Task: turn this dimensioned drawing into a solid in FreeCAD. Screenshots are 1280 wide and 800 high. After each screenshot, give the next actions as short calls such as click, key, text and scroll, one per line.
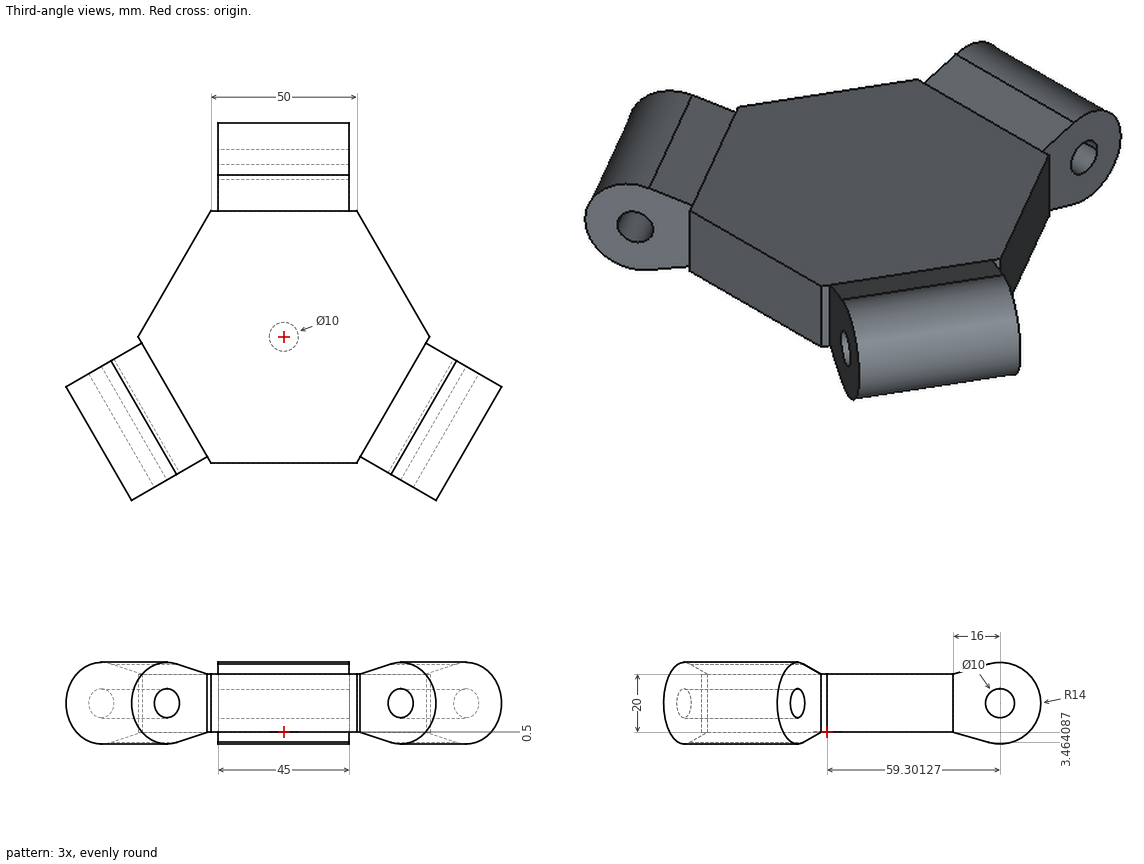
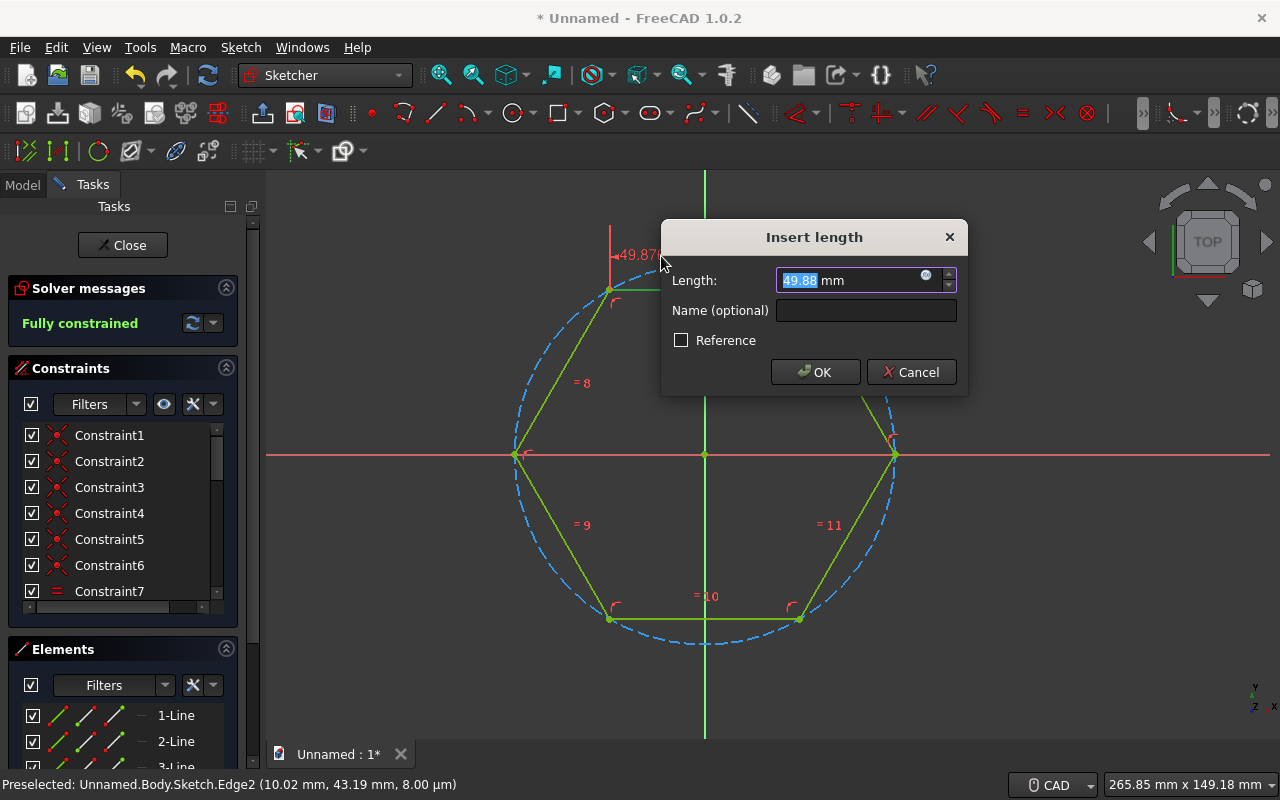
text(50)
key(Return)
key(Escape)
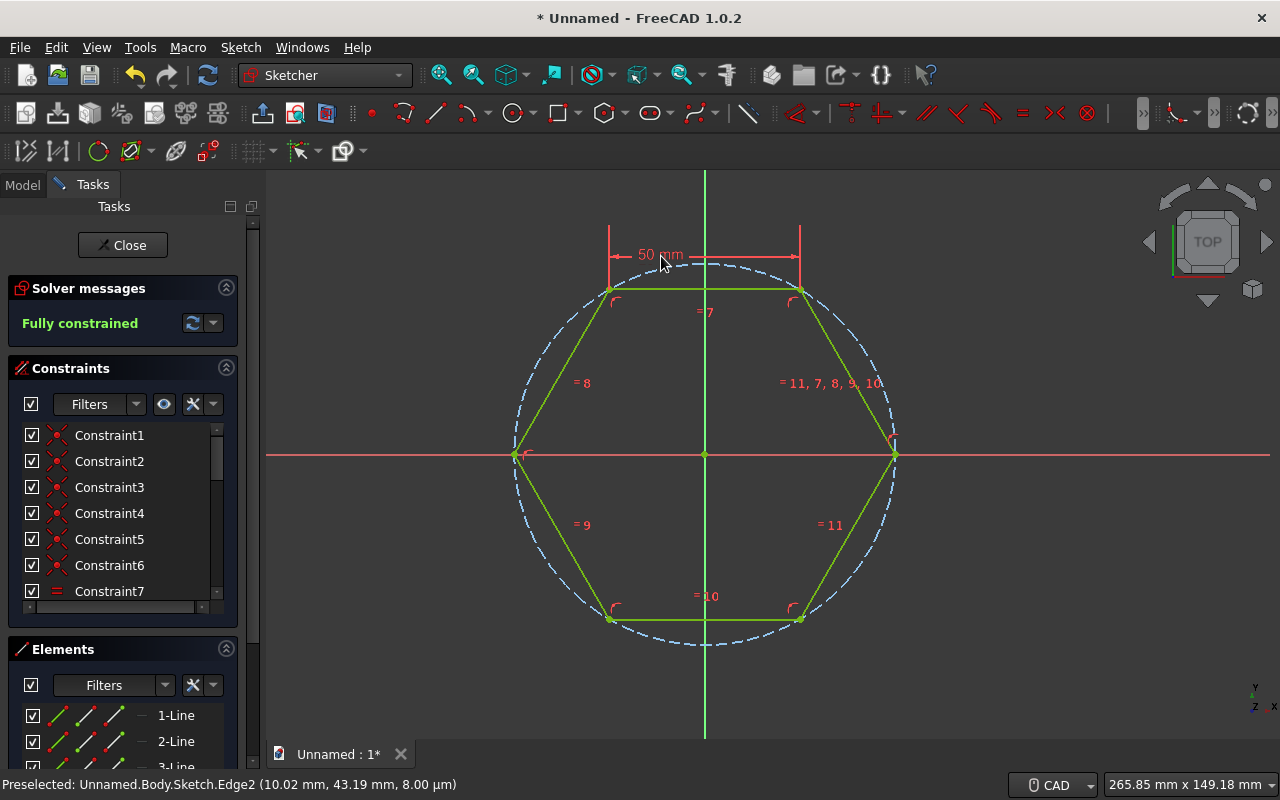
click(123, 245)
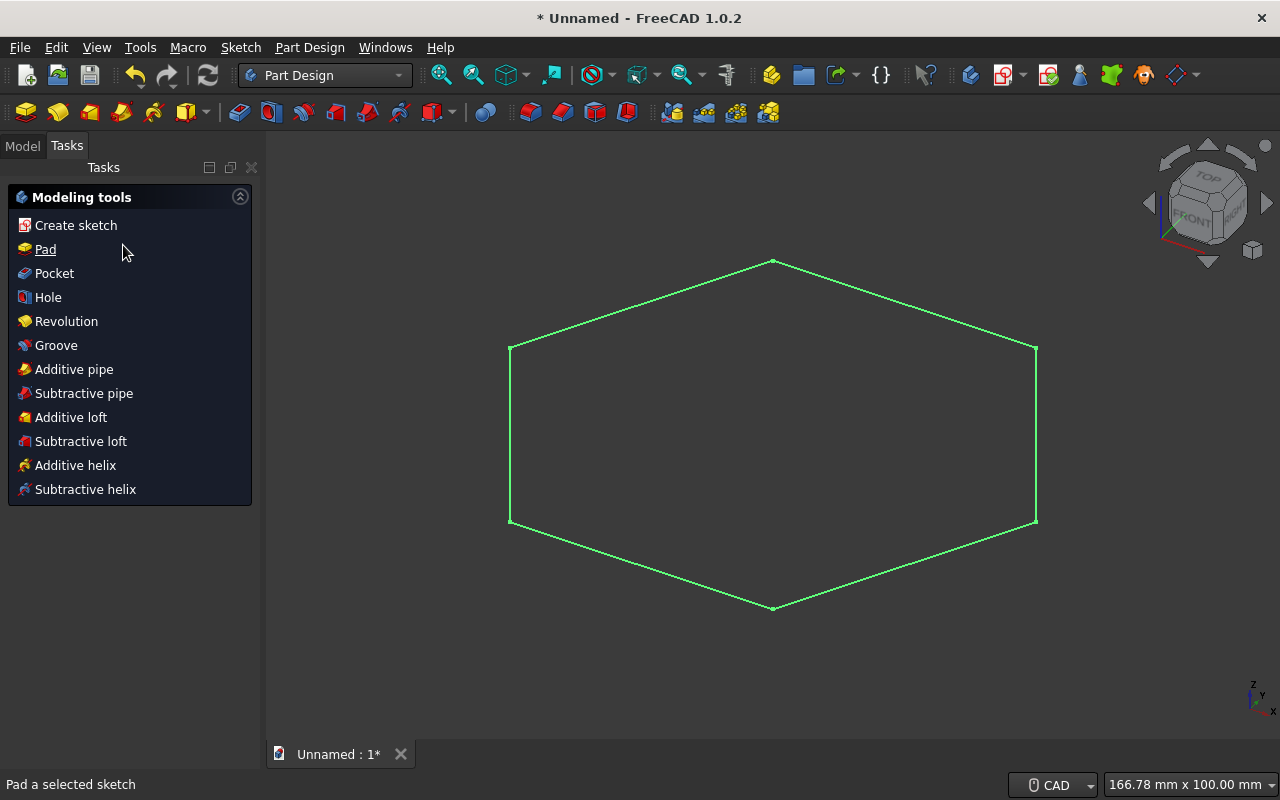
click(26, 112)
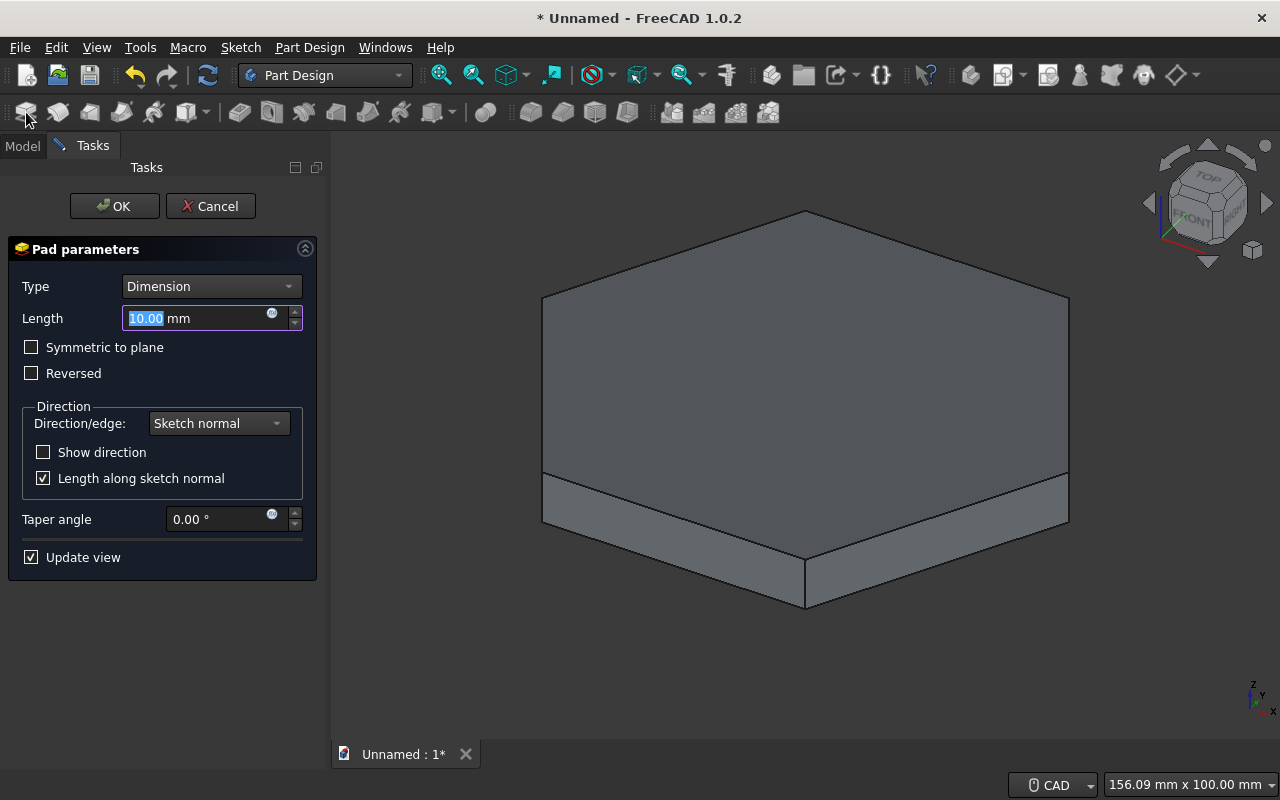
text(20)
key(Tab)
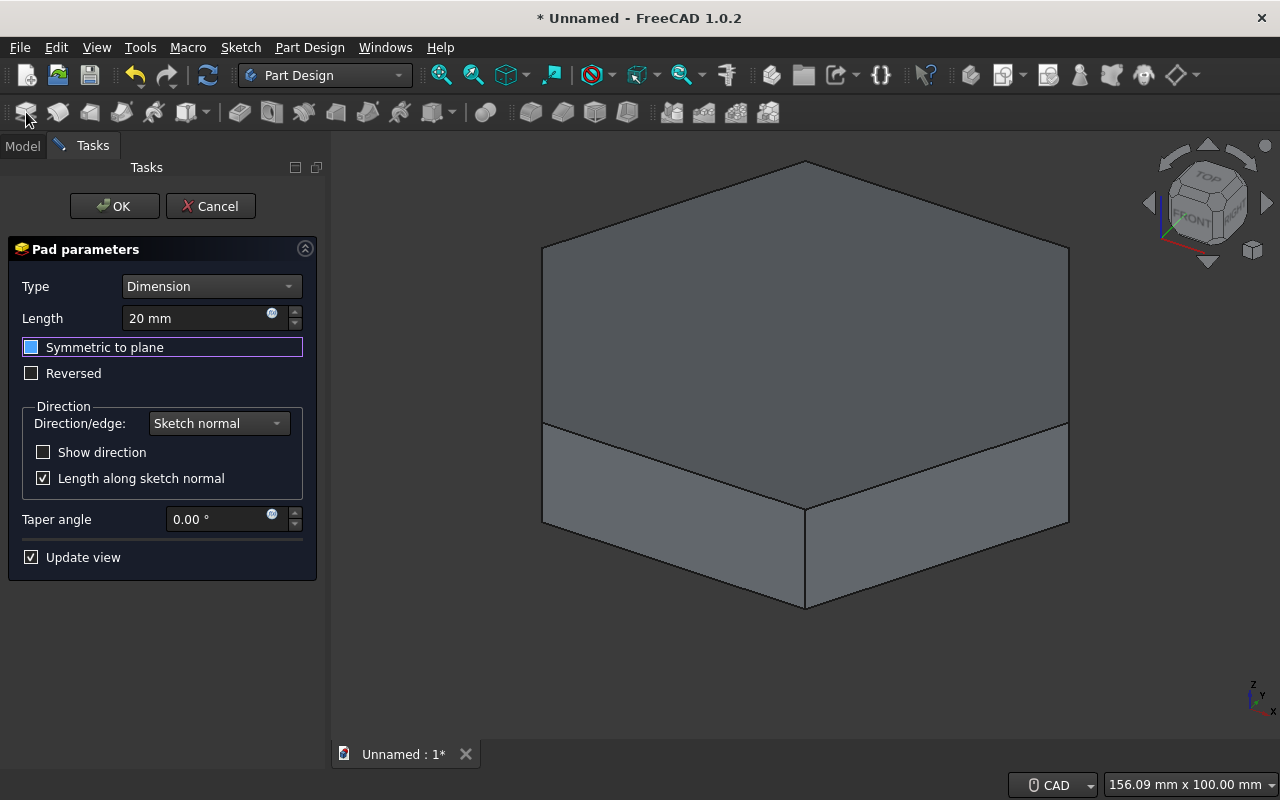
click(115, 206)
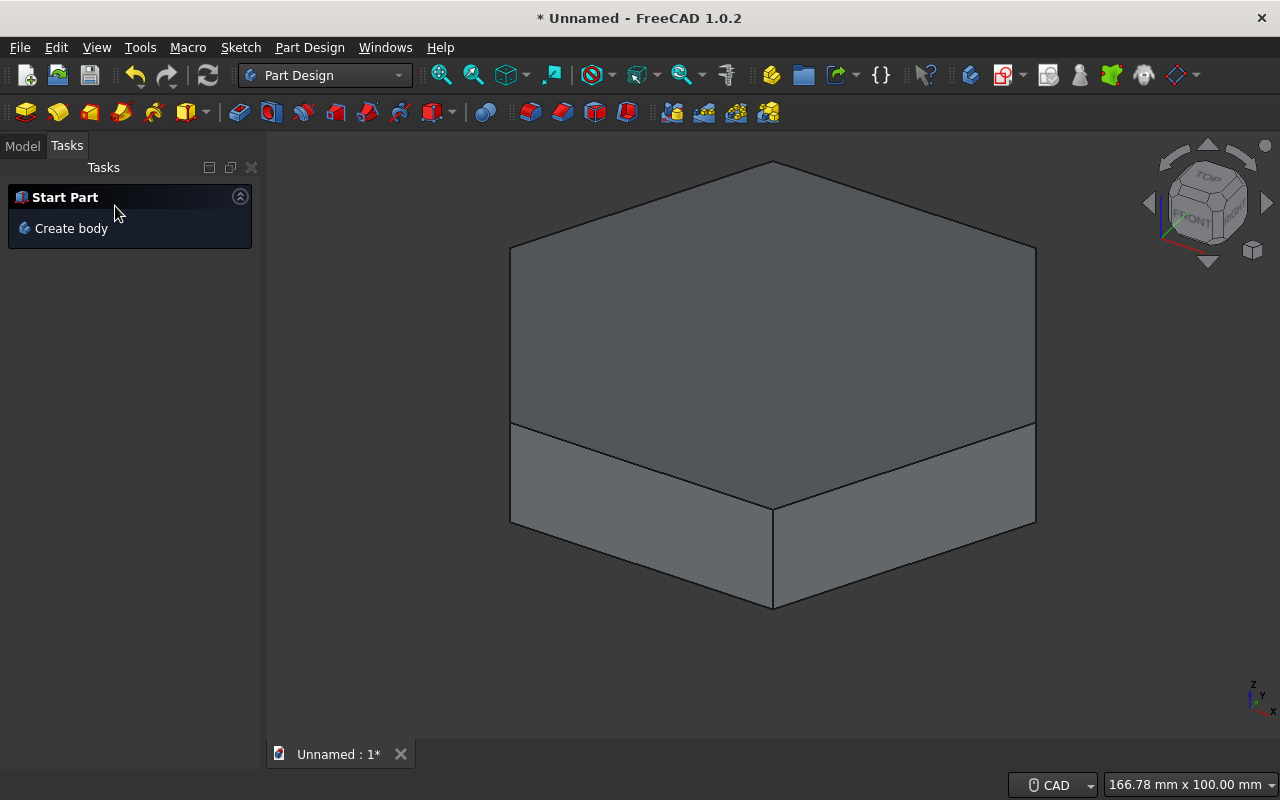
click(442, 76)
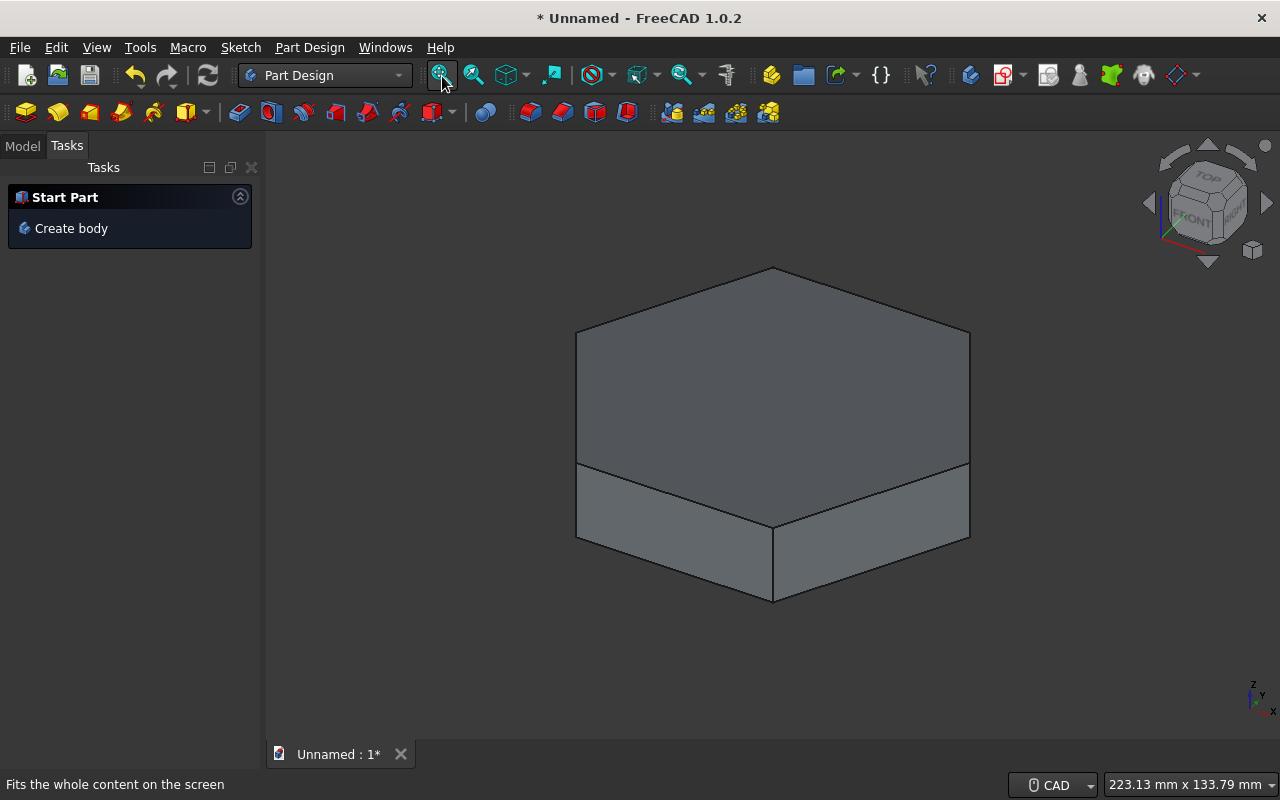
click(1004, 76)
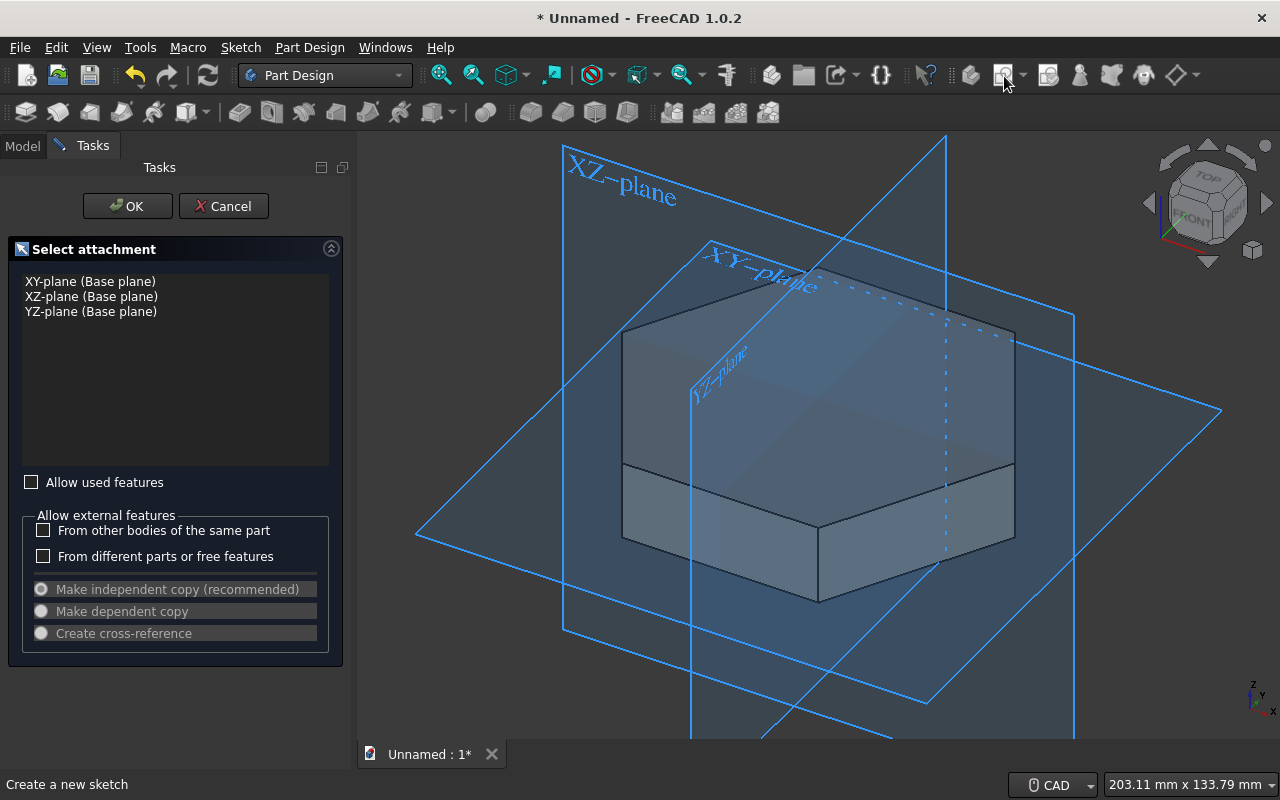
click(82, 312)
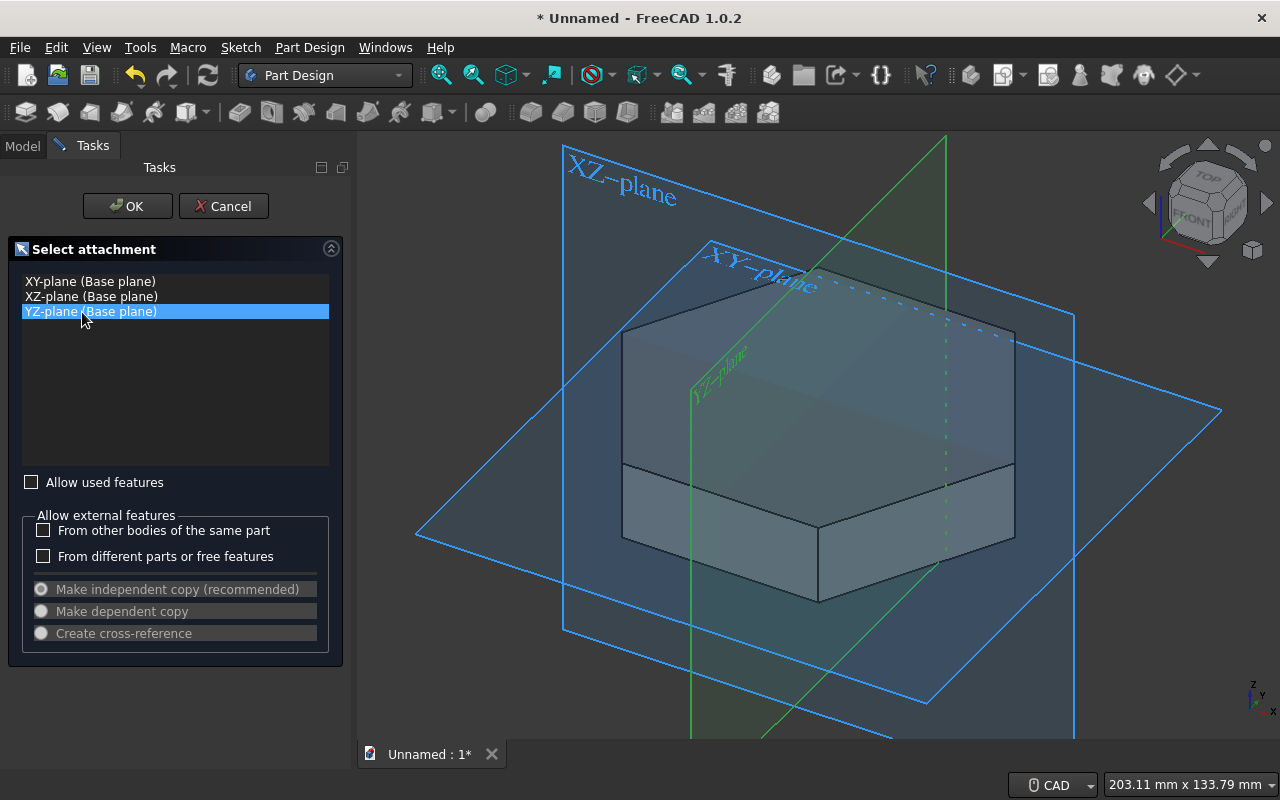
click(128, 206)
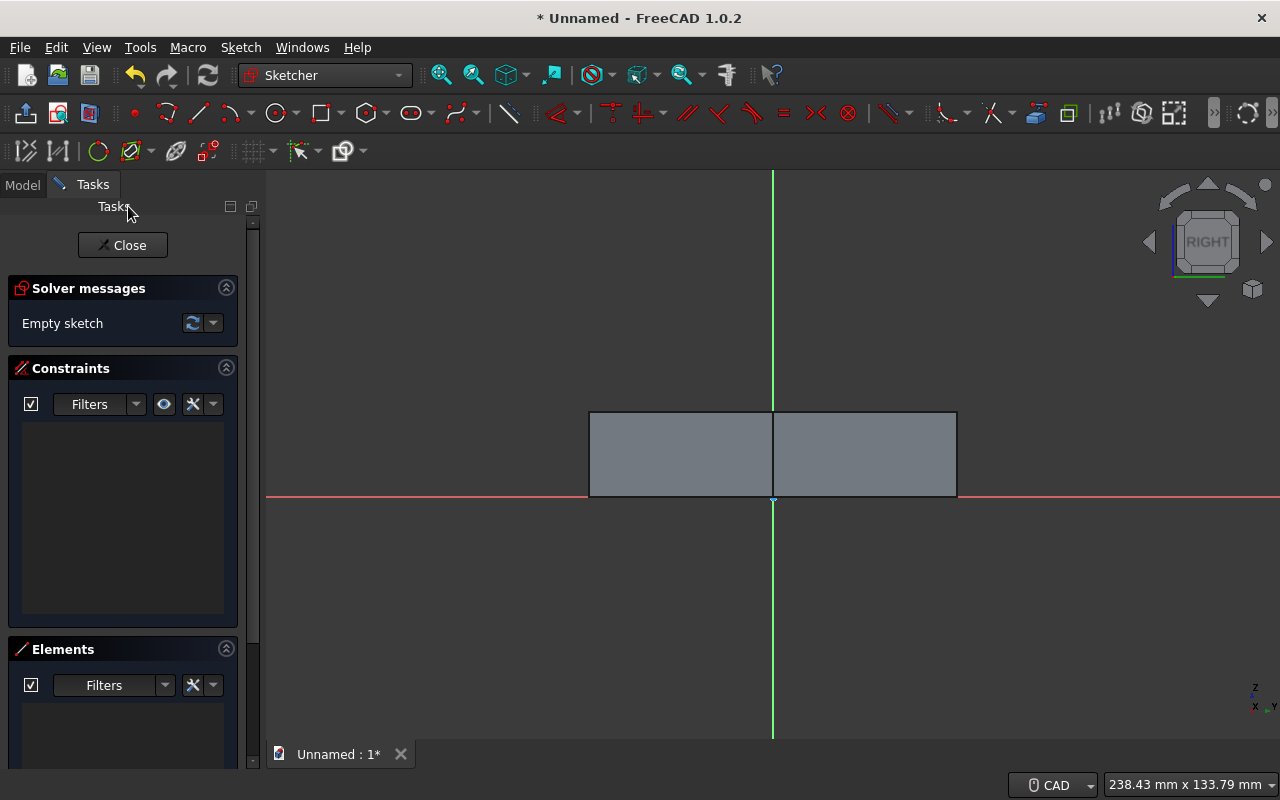
click(90, 114)